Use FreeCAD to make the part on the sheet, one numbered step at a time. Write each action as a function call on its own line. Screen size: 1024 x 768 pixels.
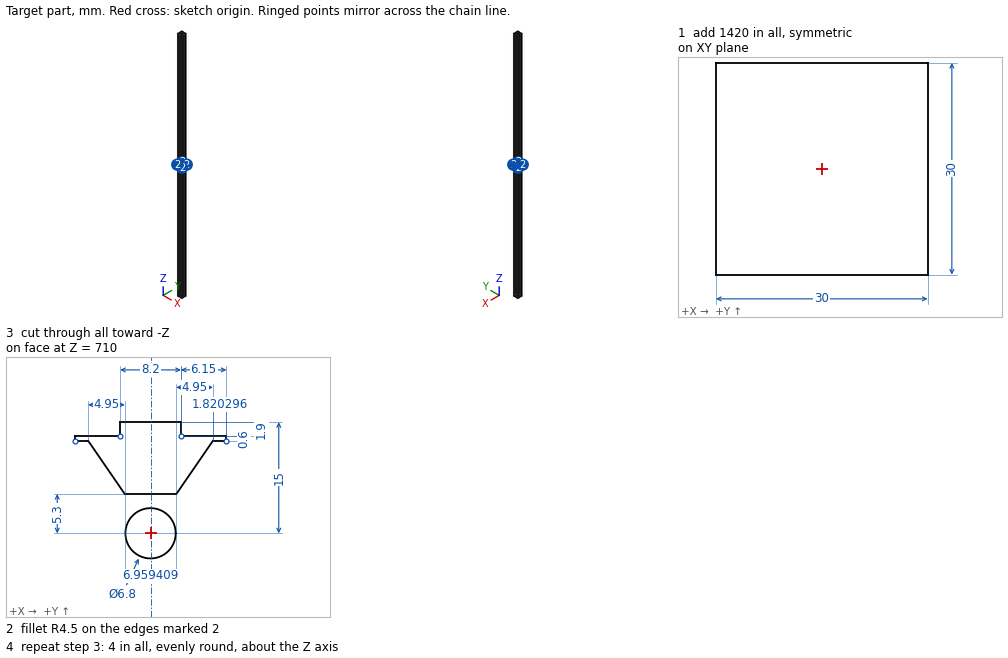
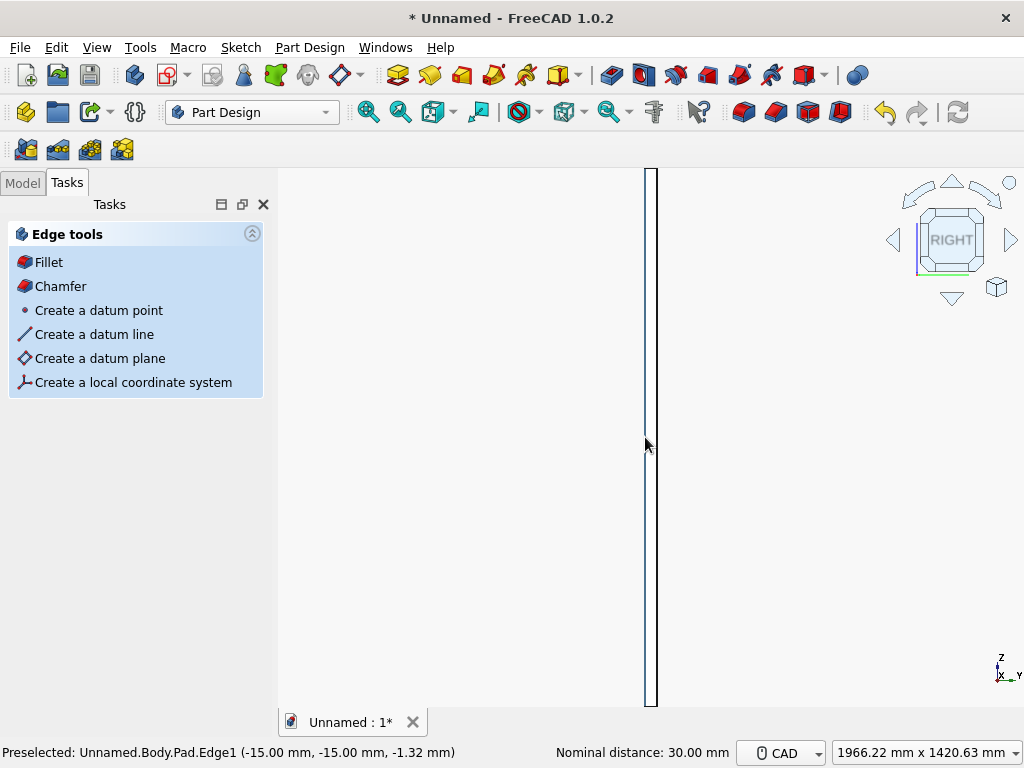
key(v)
key(f)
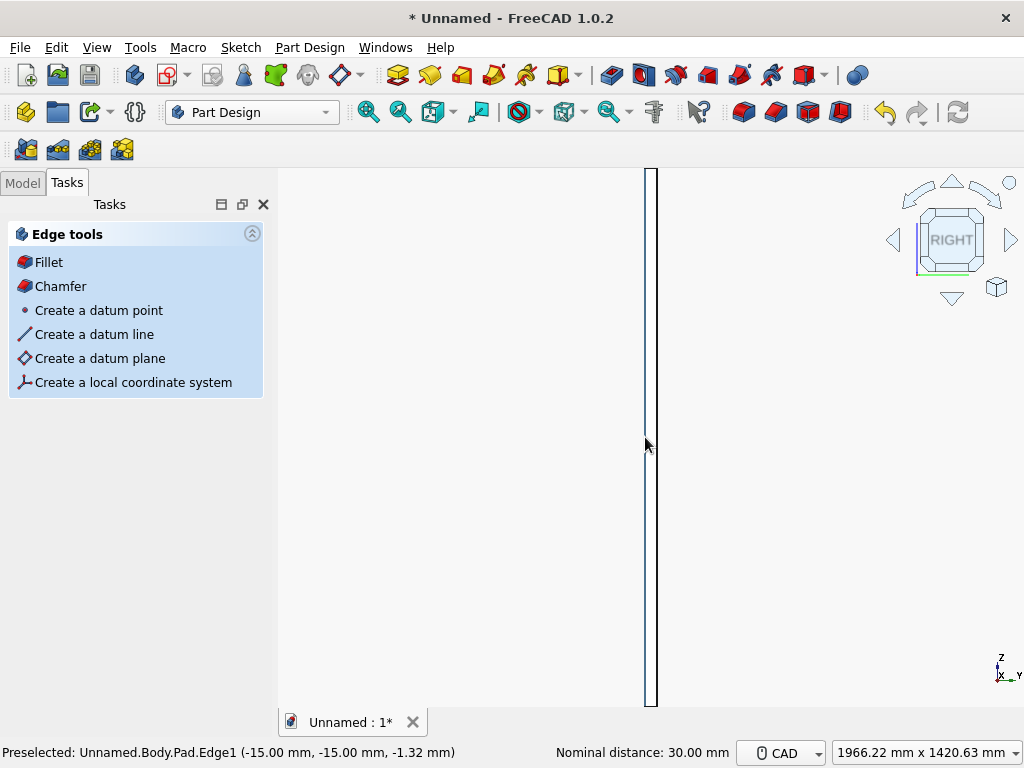
click(657, 436, ctrl)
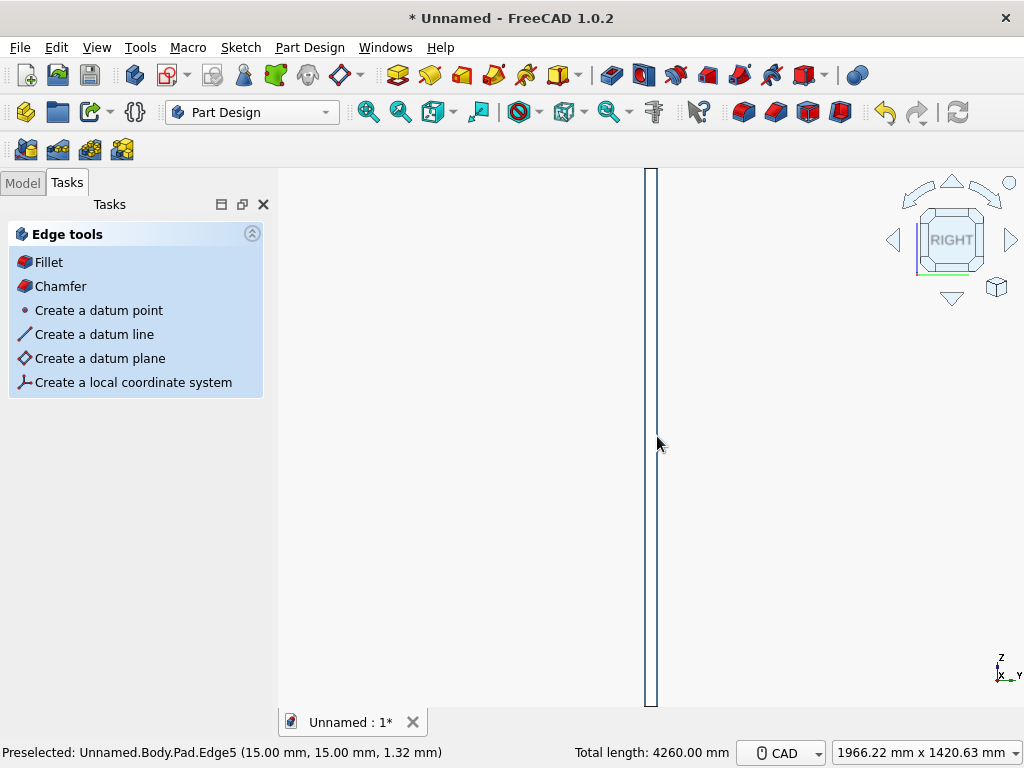
key(5)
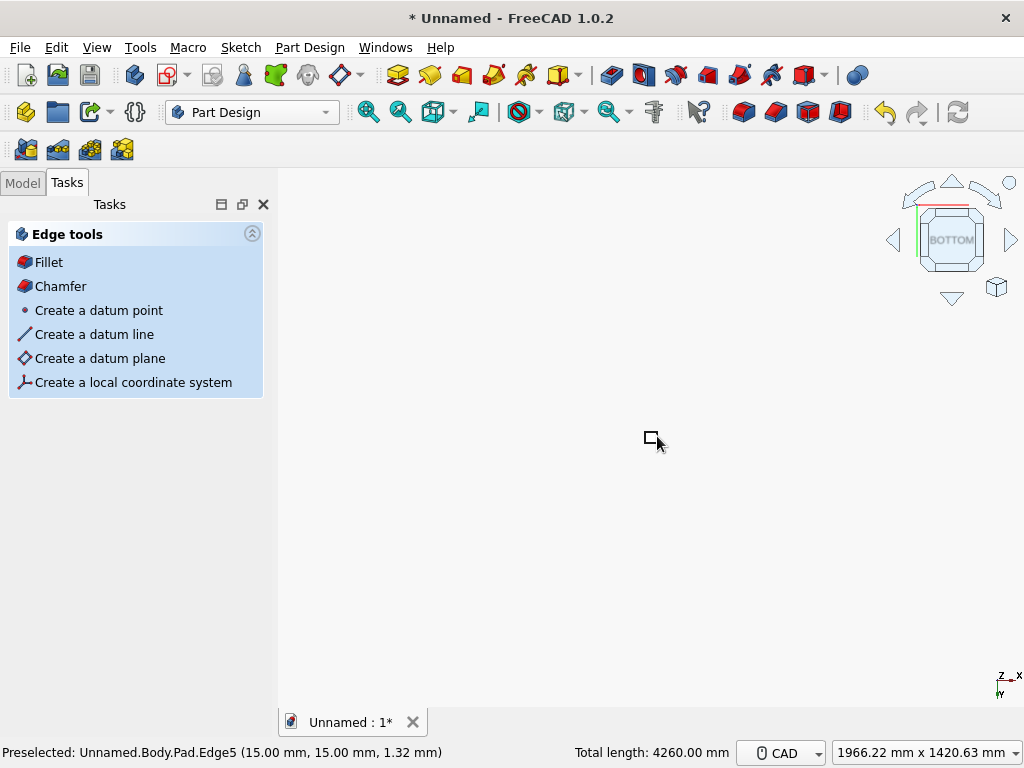
key(v)
key(f)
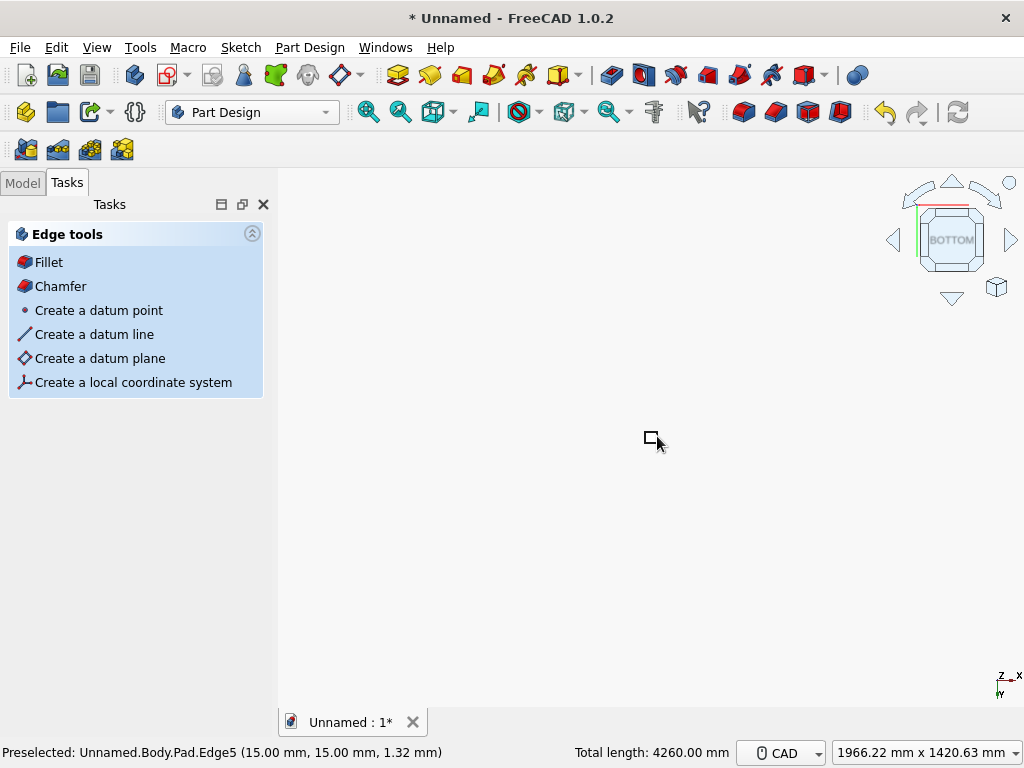
key(4)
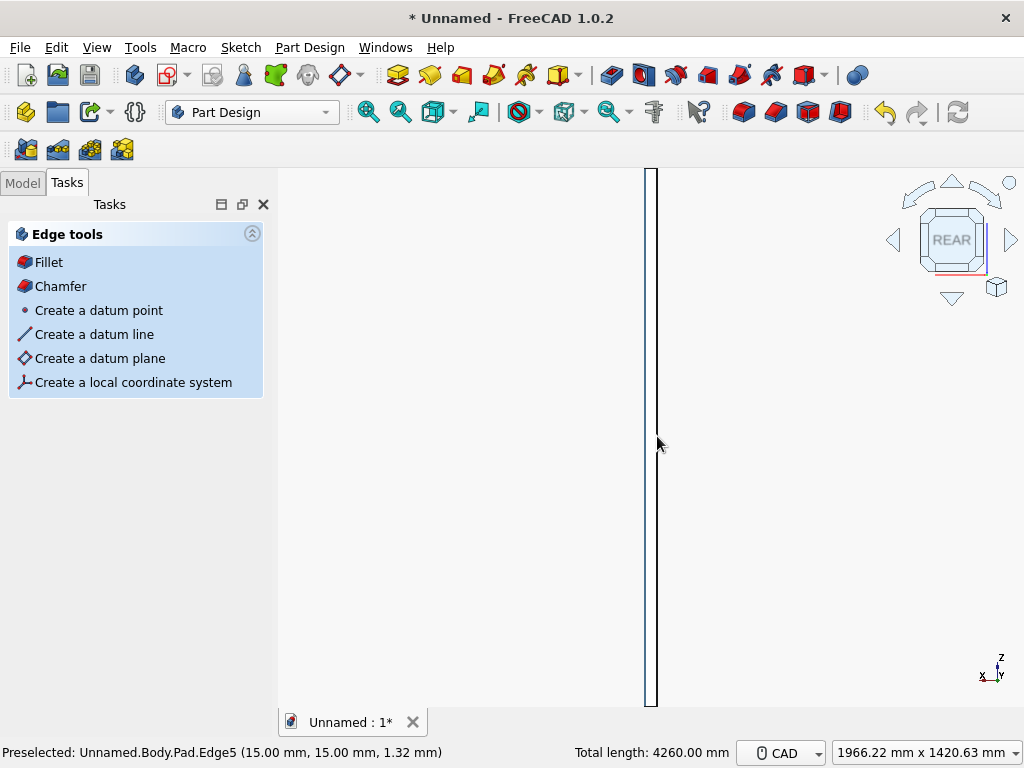
click(370, 112)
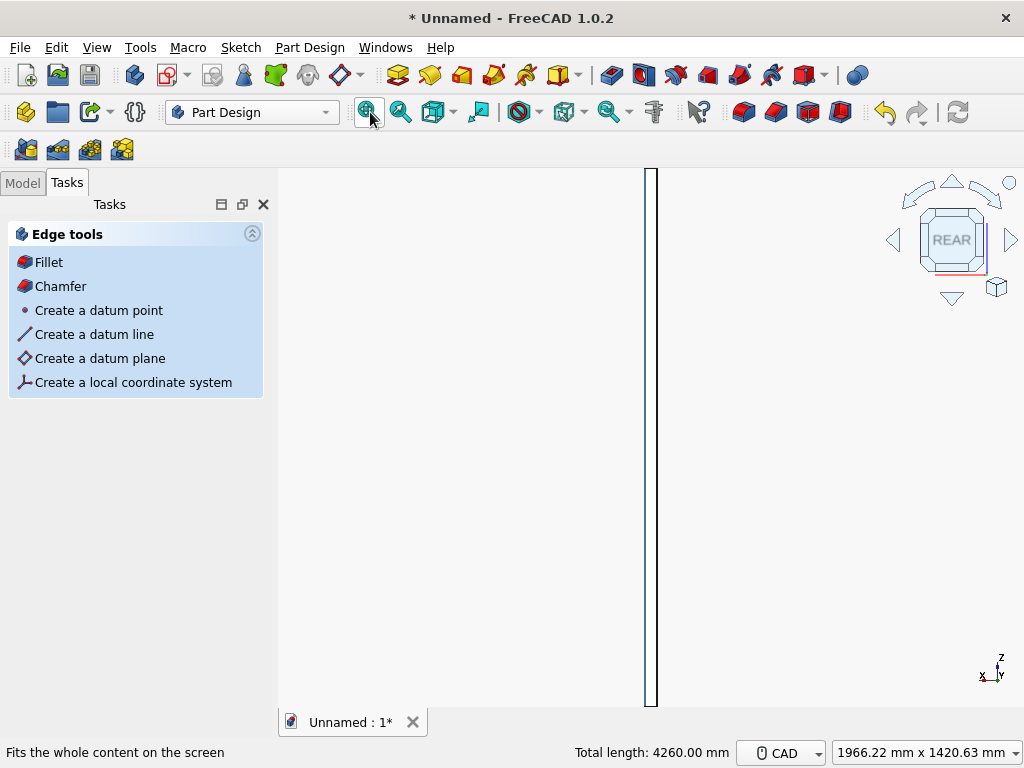
click(657, 437, ctrl)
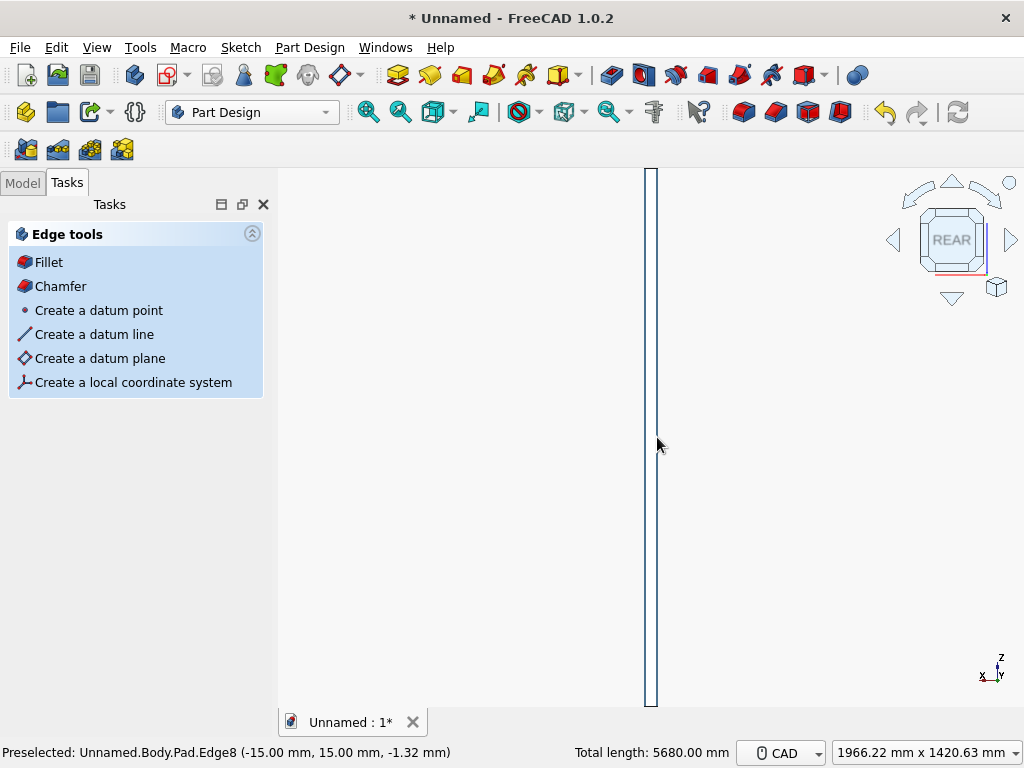
click(744, 112)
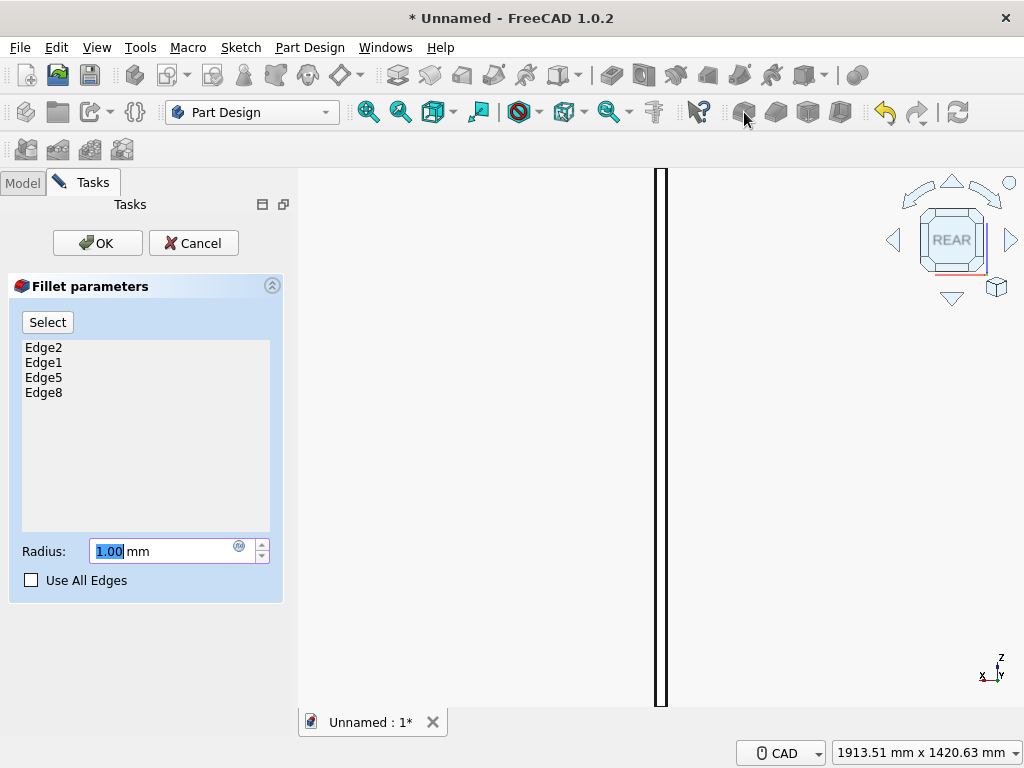
text(4.5)
key(Tab)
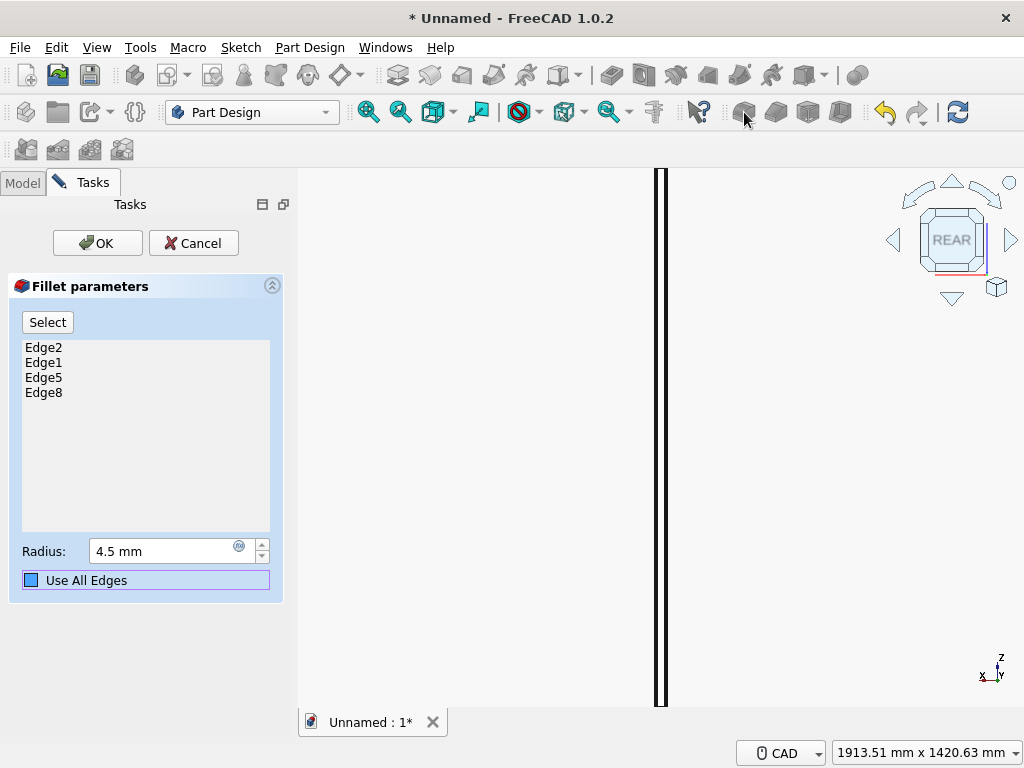
click(98, 243)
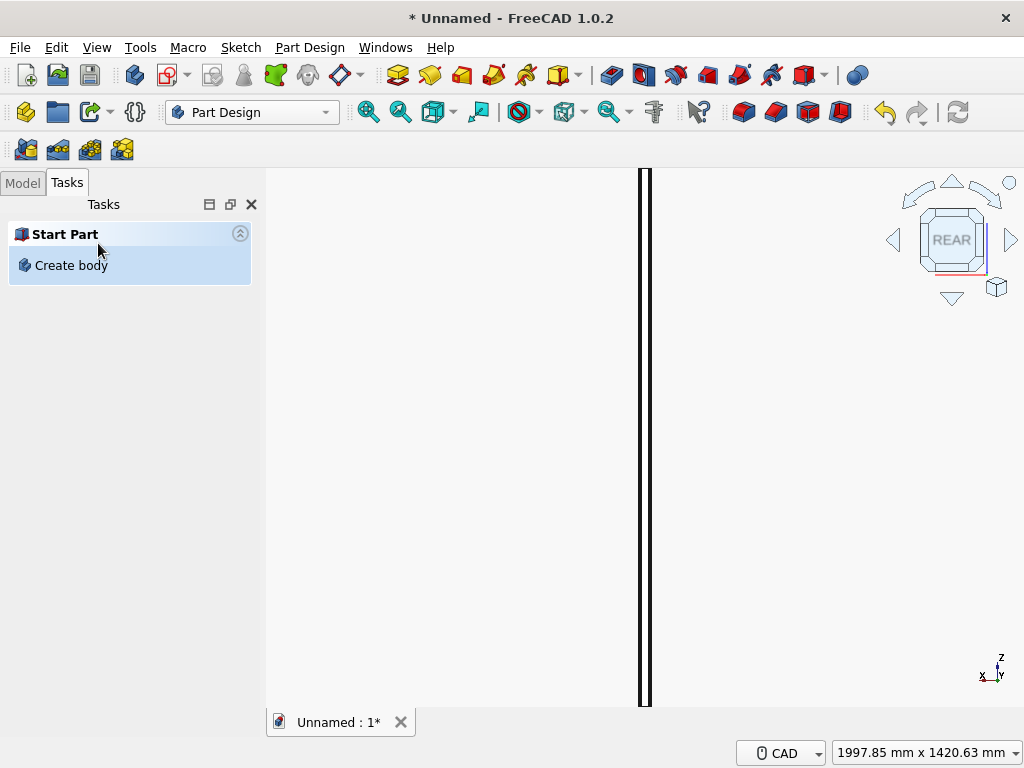
key(v)
key(f)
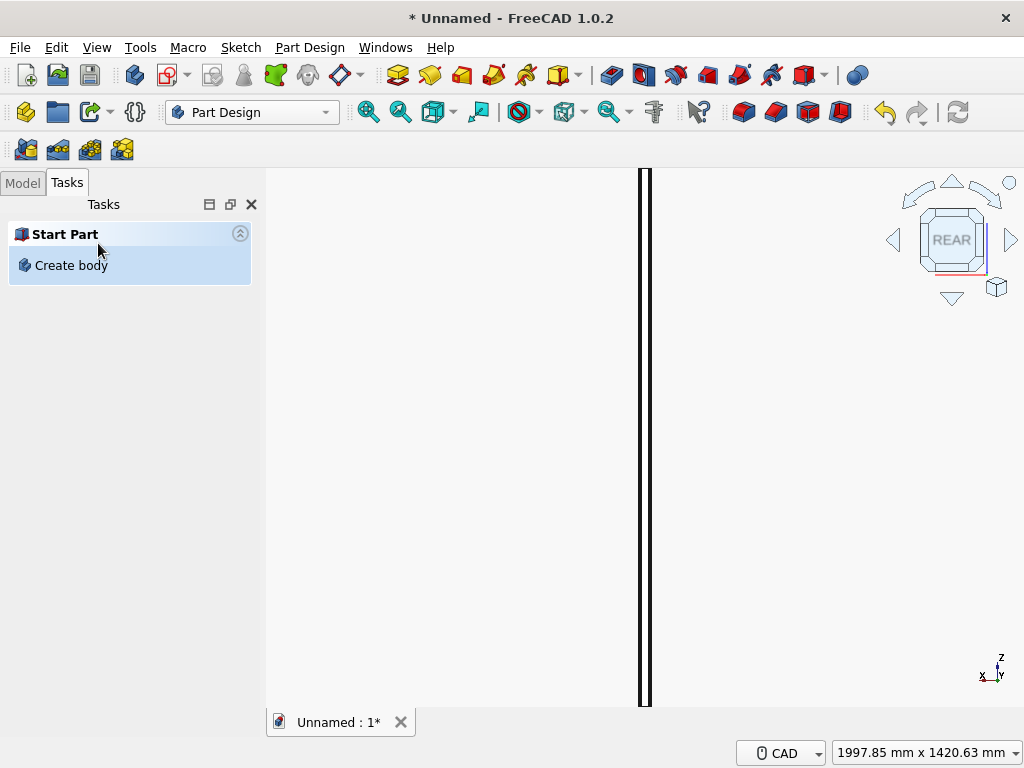
key(0)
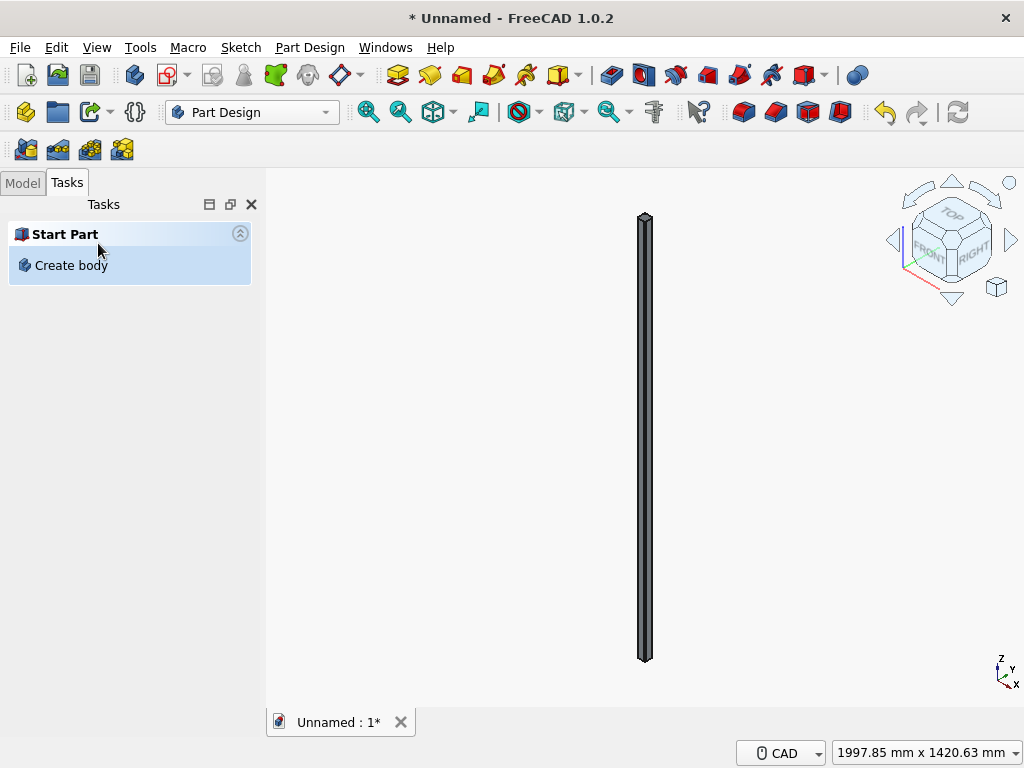
scroll(645, 217, up, 4)